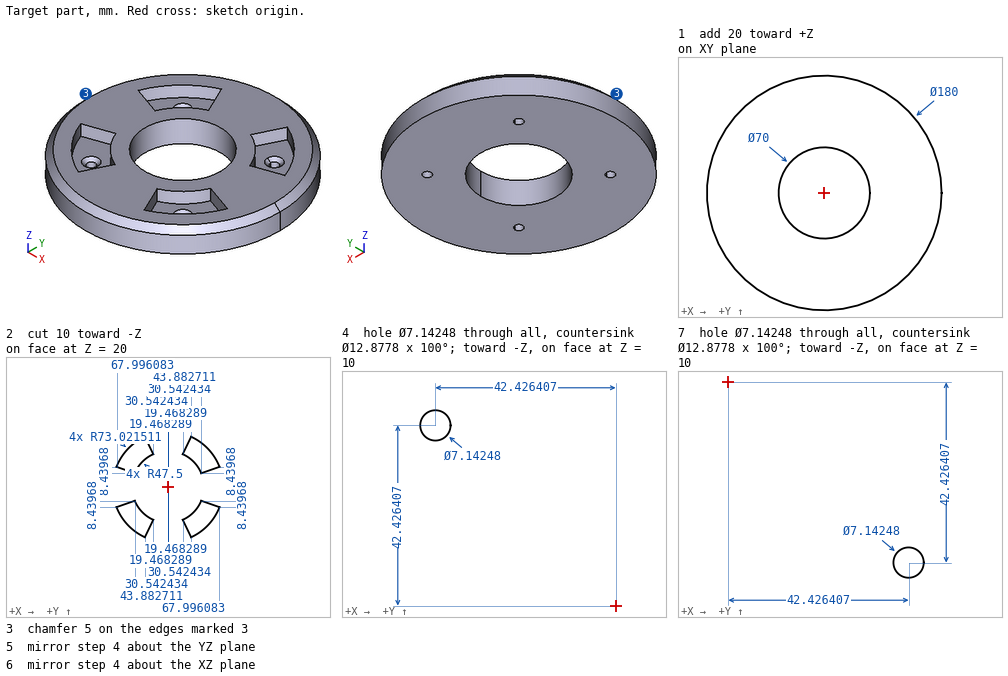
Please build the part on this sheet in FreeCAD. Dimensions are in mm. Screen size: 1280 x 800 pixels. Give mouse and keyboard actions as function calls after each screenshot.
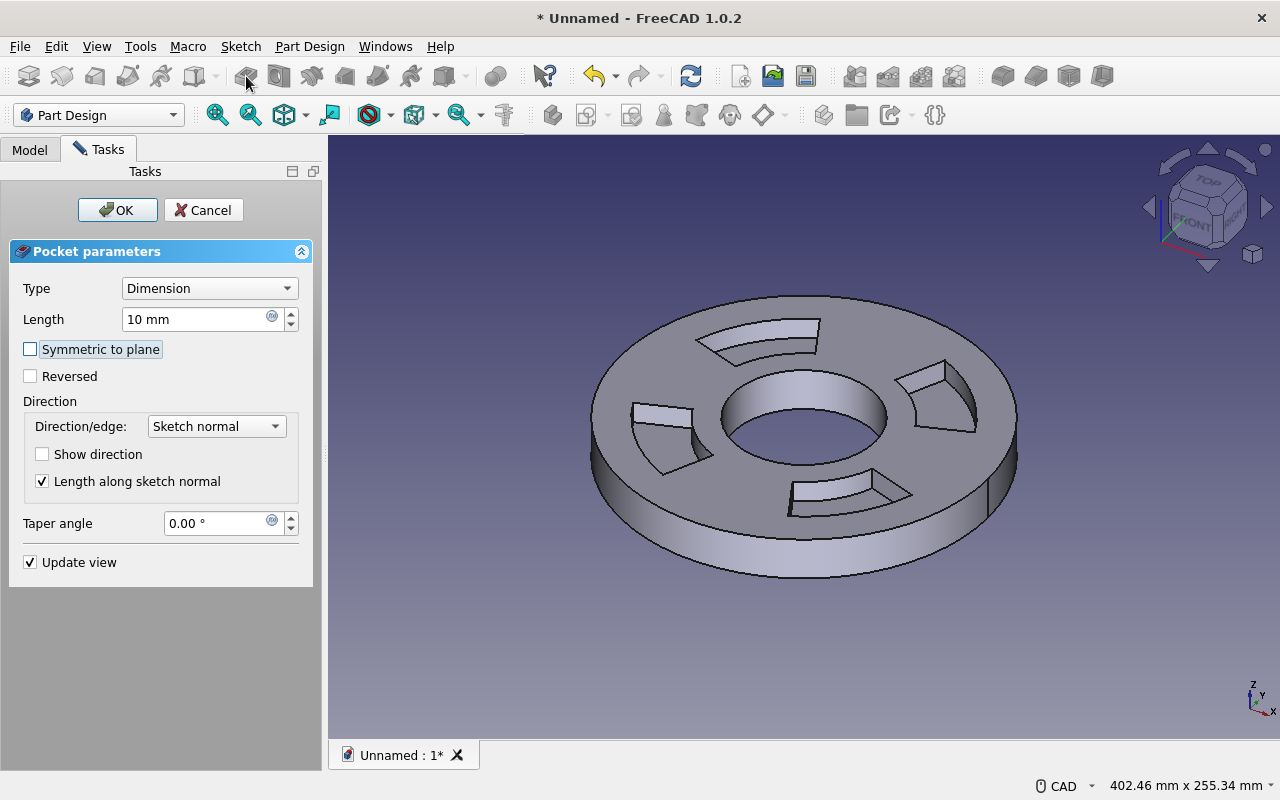
click(118, 210)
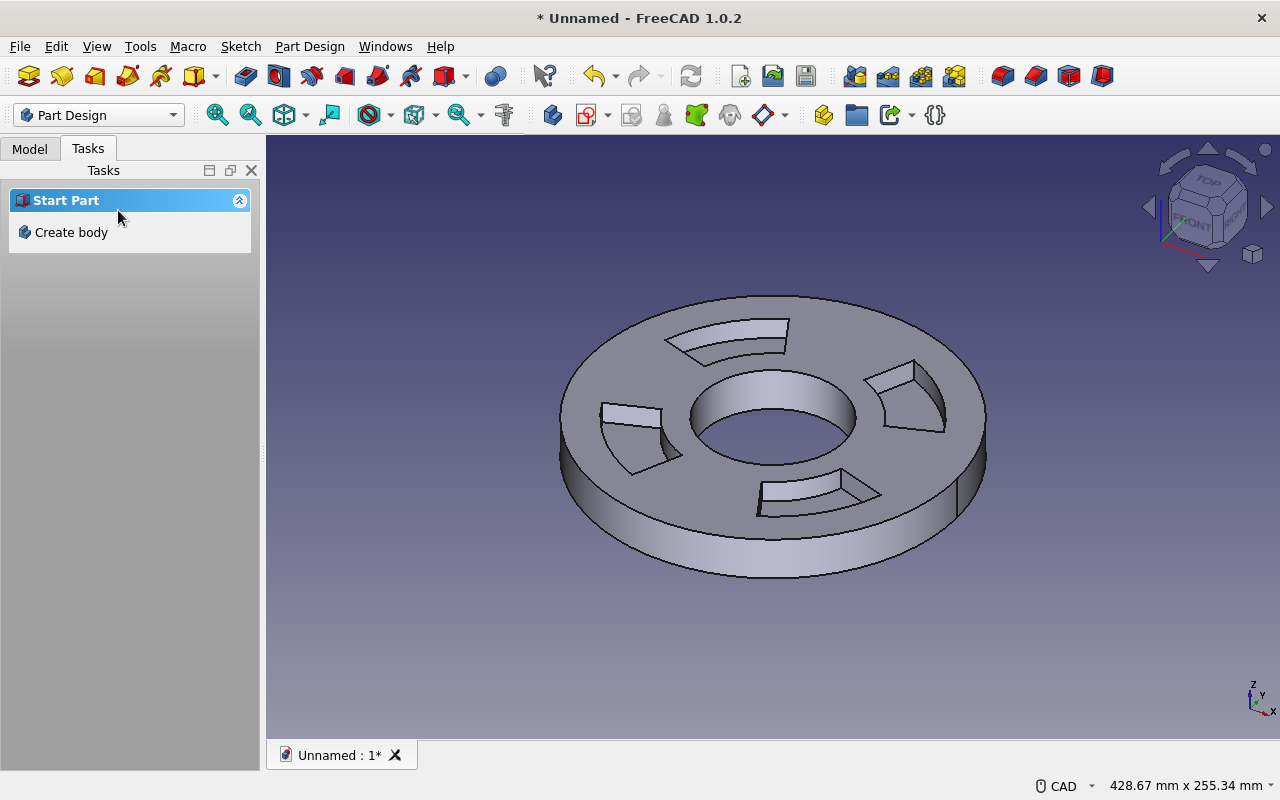
click(561, 429)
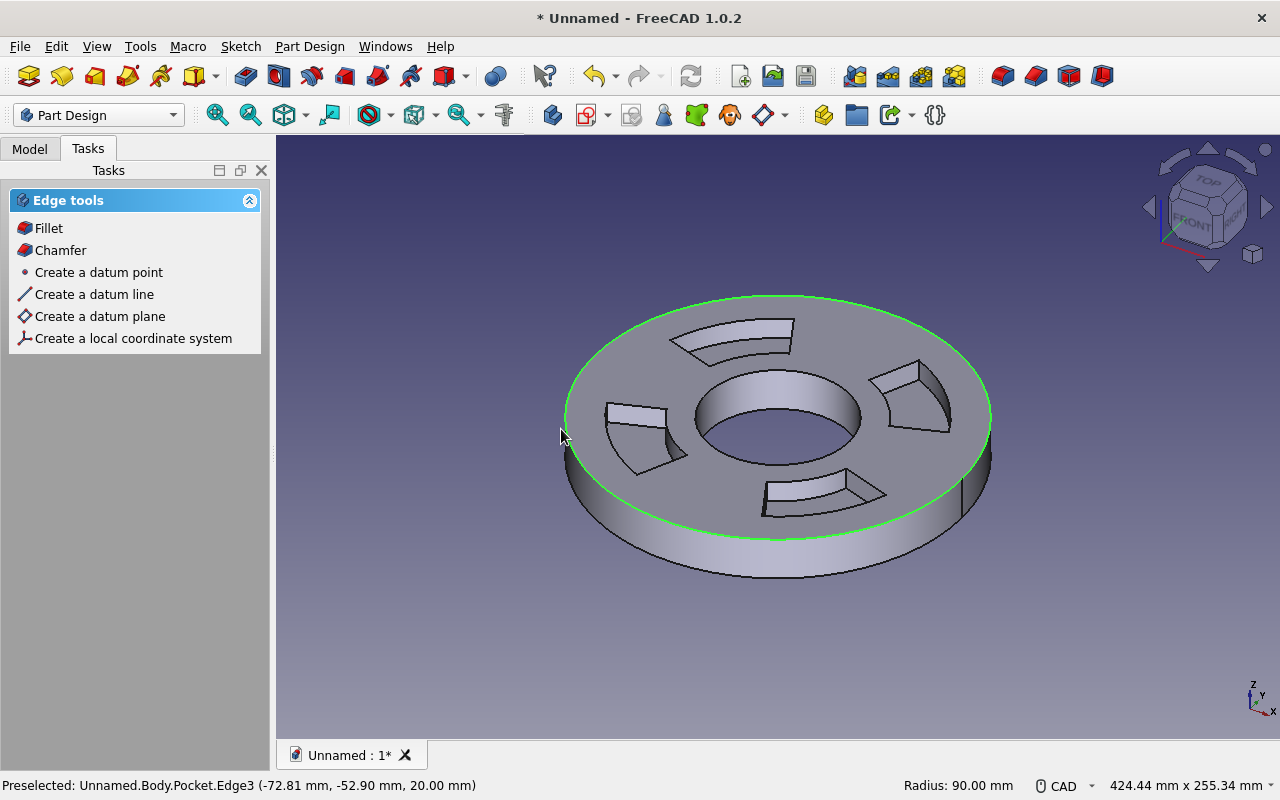
click(1036, 76)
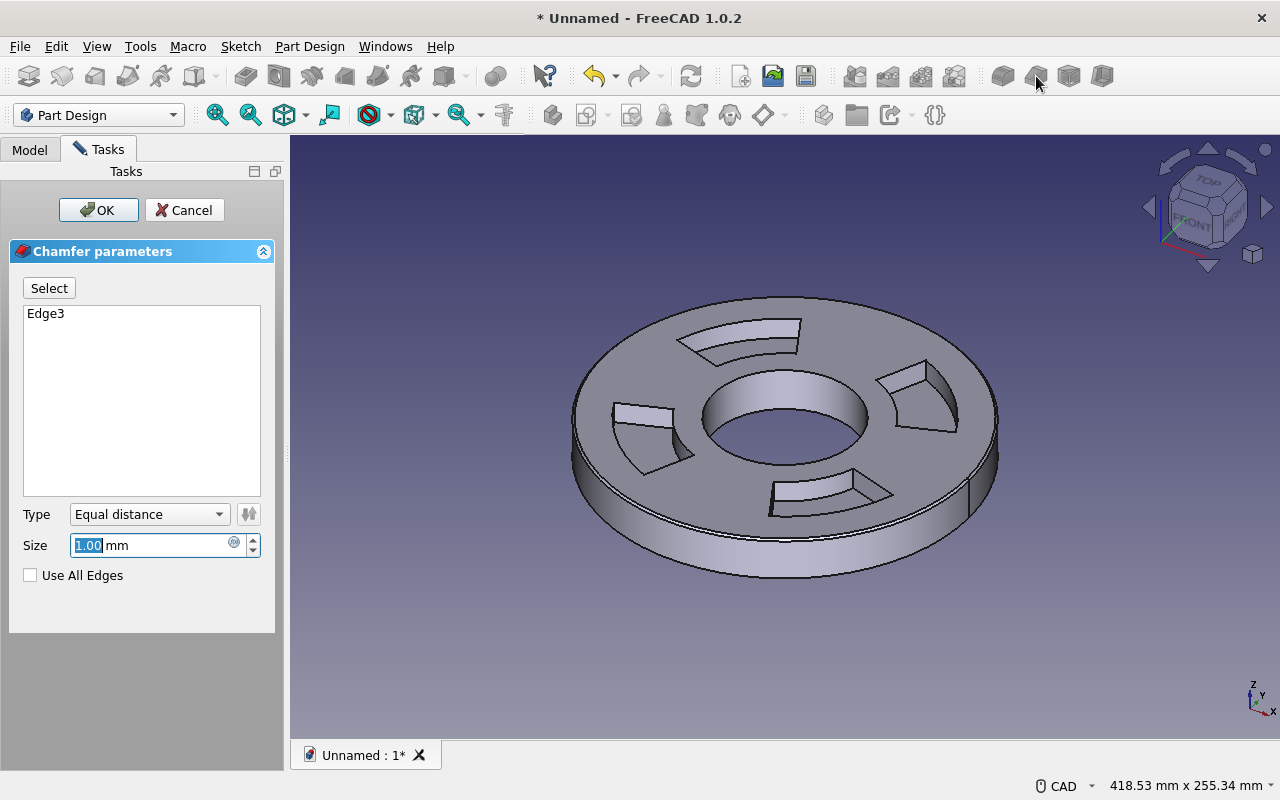
text(5)
key(Tab)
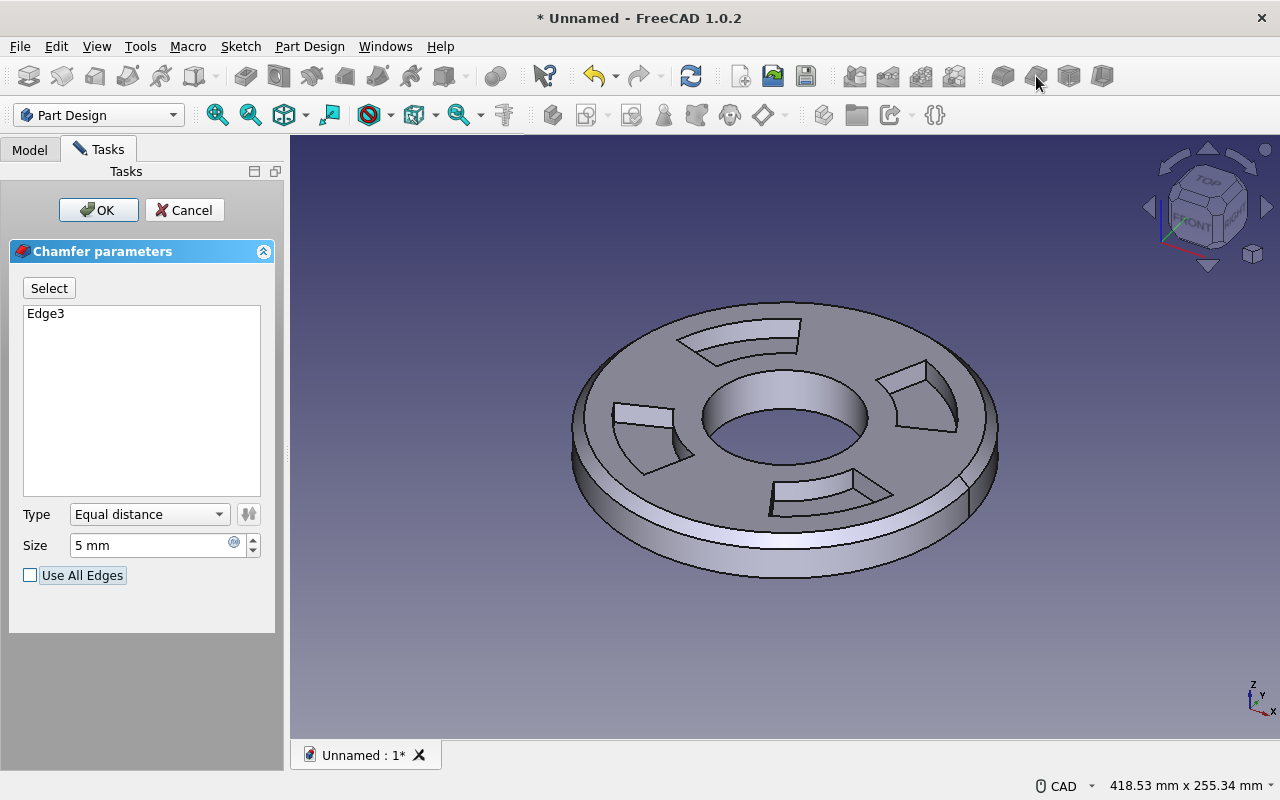
click(99, 210)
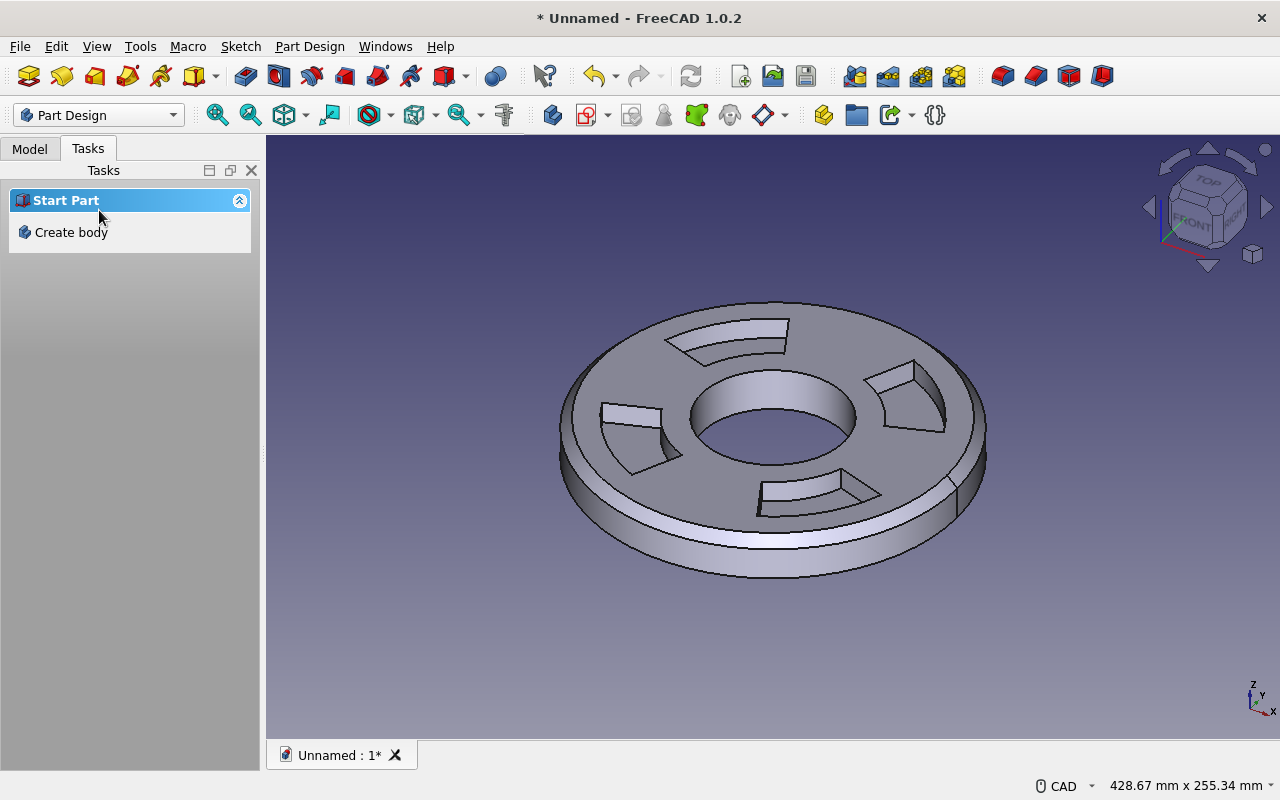
click(633, 456)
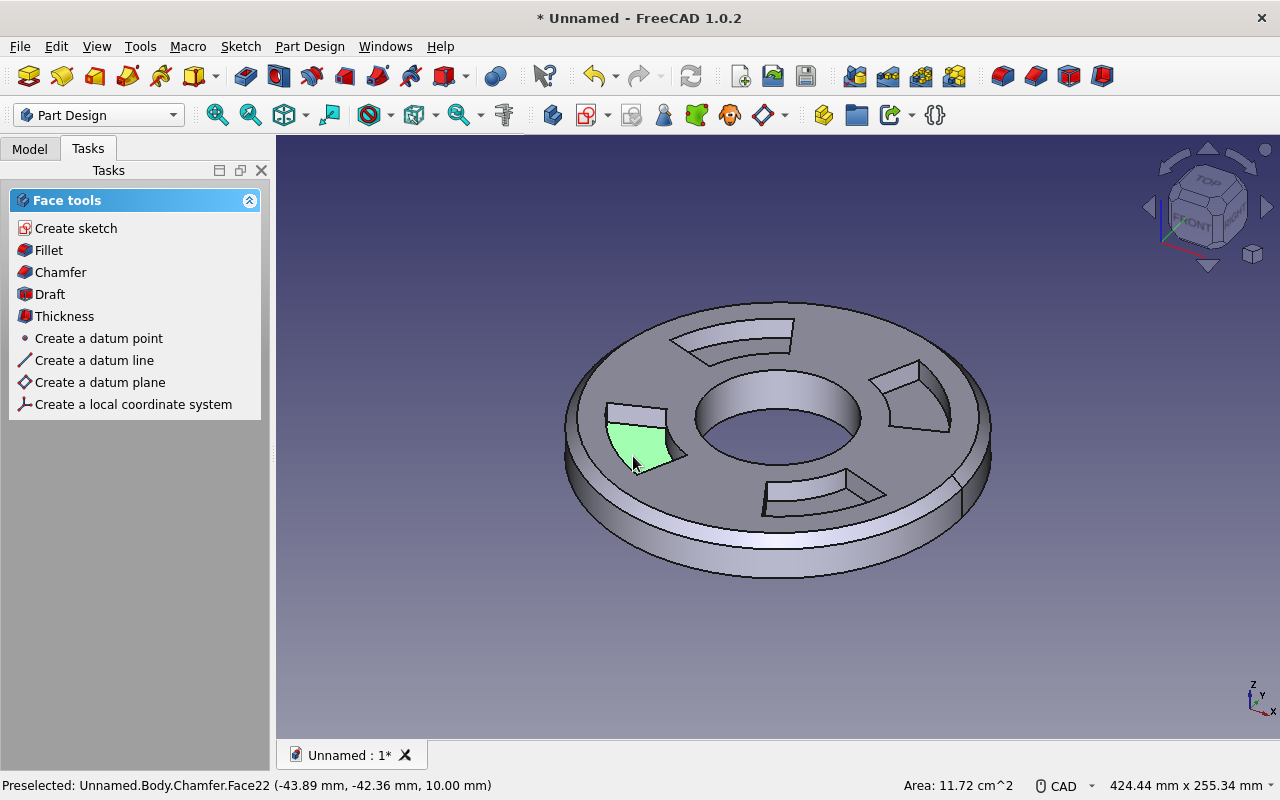
click(586, 116)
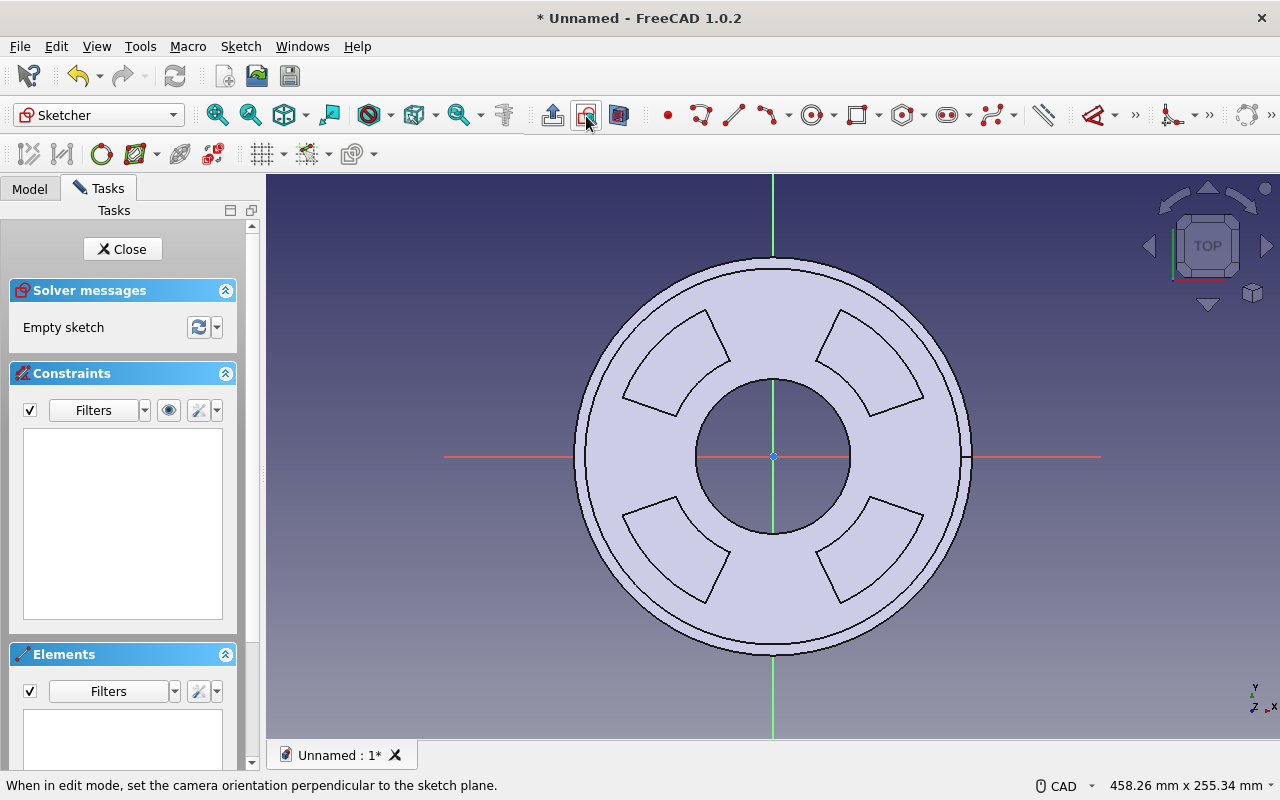
key(q)
key(s)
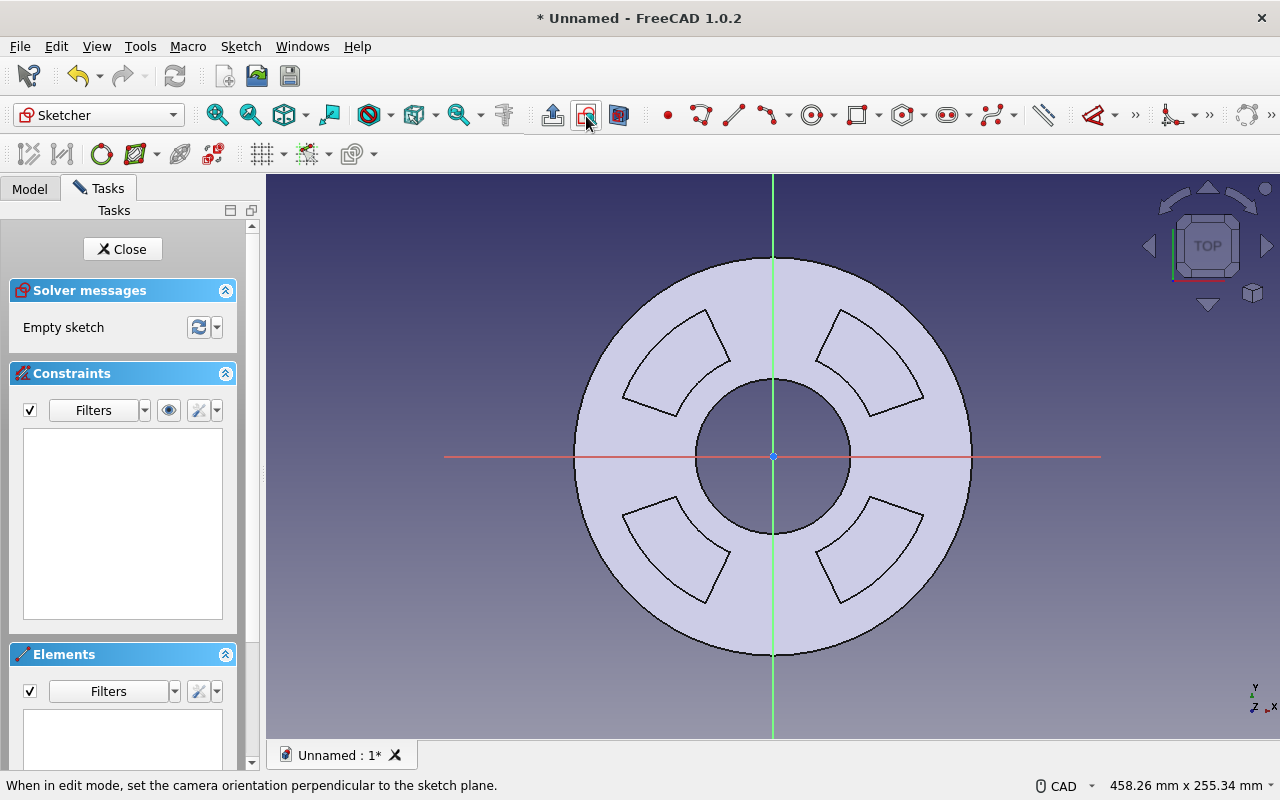
scroll(678, 358, up, 15)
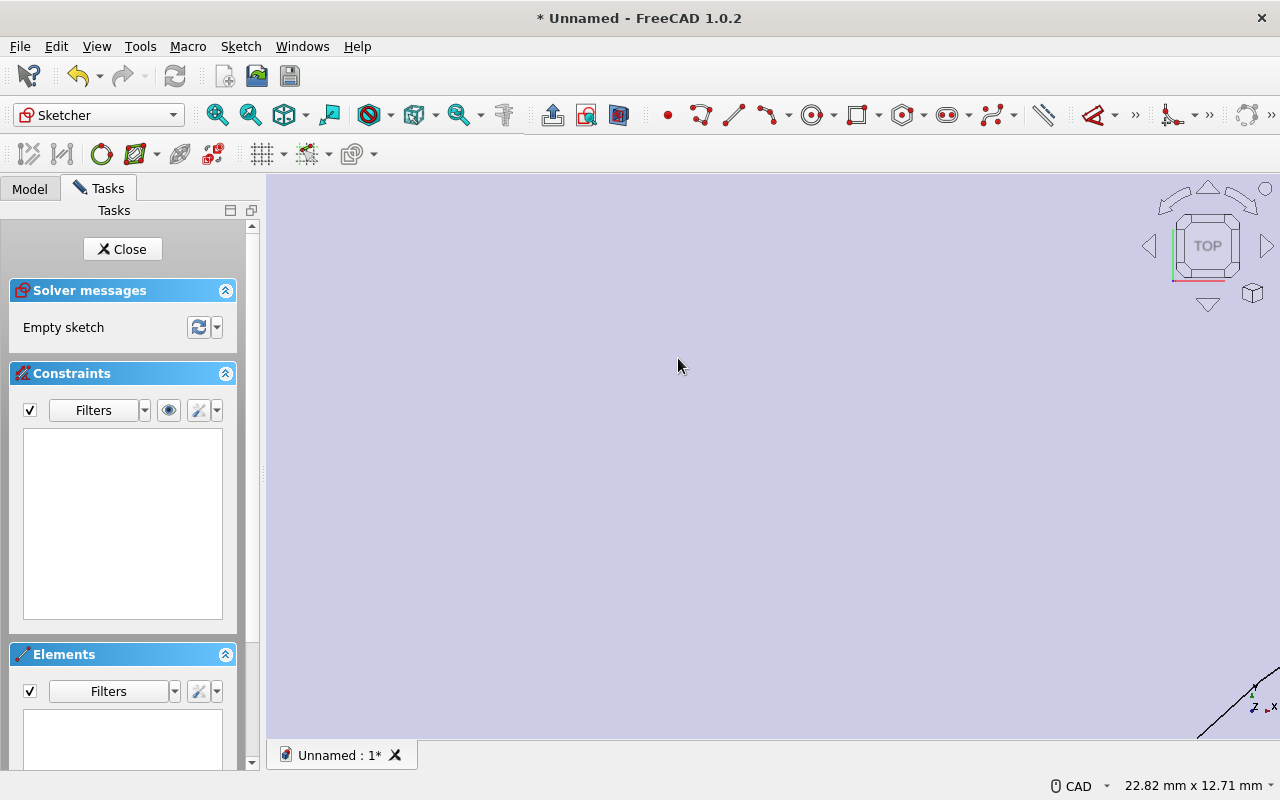
click(812, 116)